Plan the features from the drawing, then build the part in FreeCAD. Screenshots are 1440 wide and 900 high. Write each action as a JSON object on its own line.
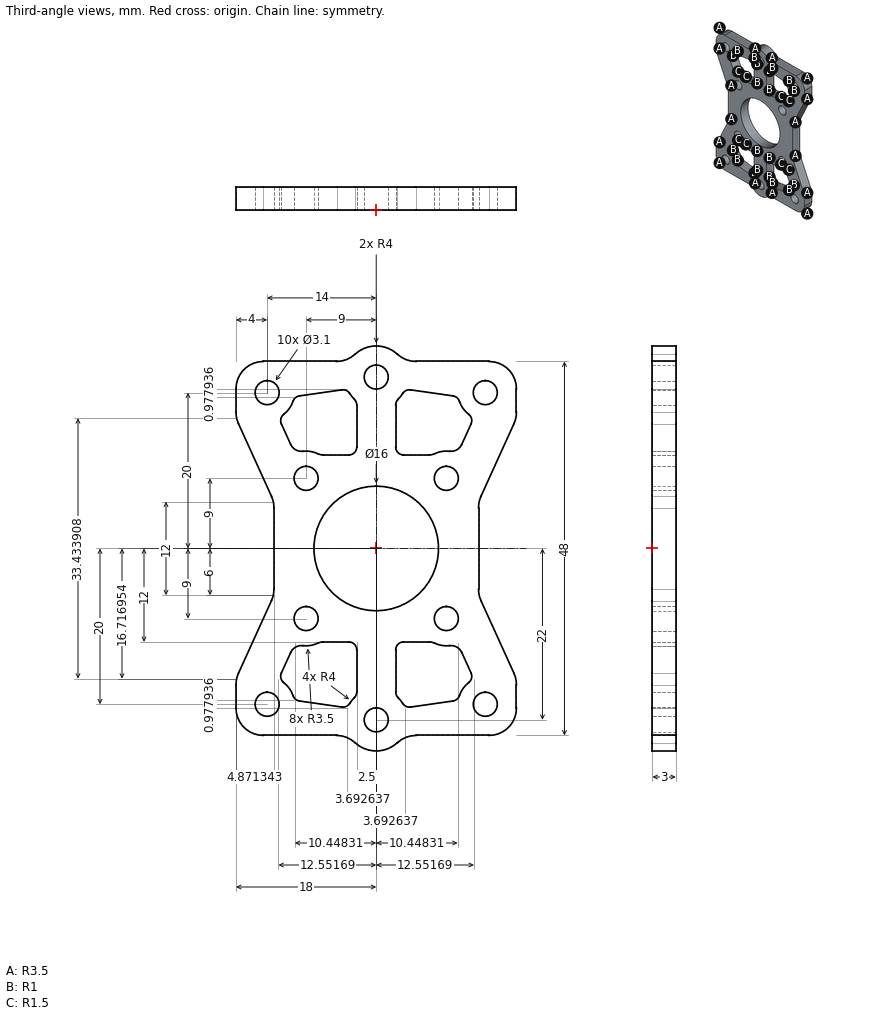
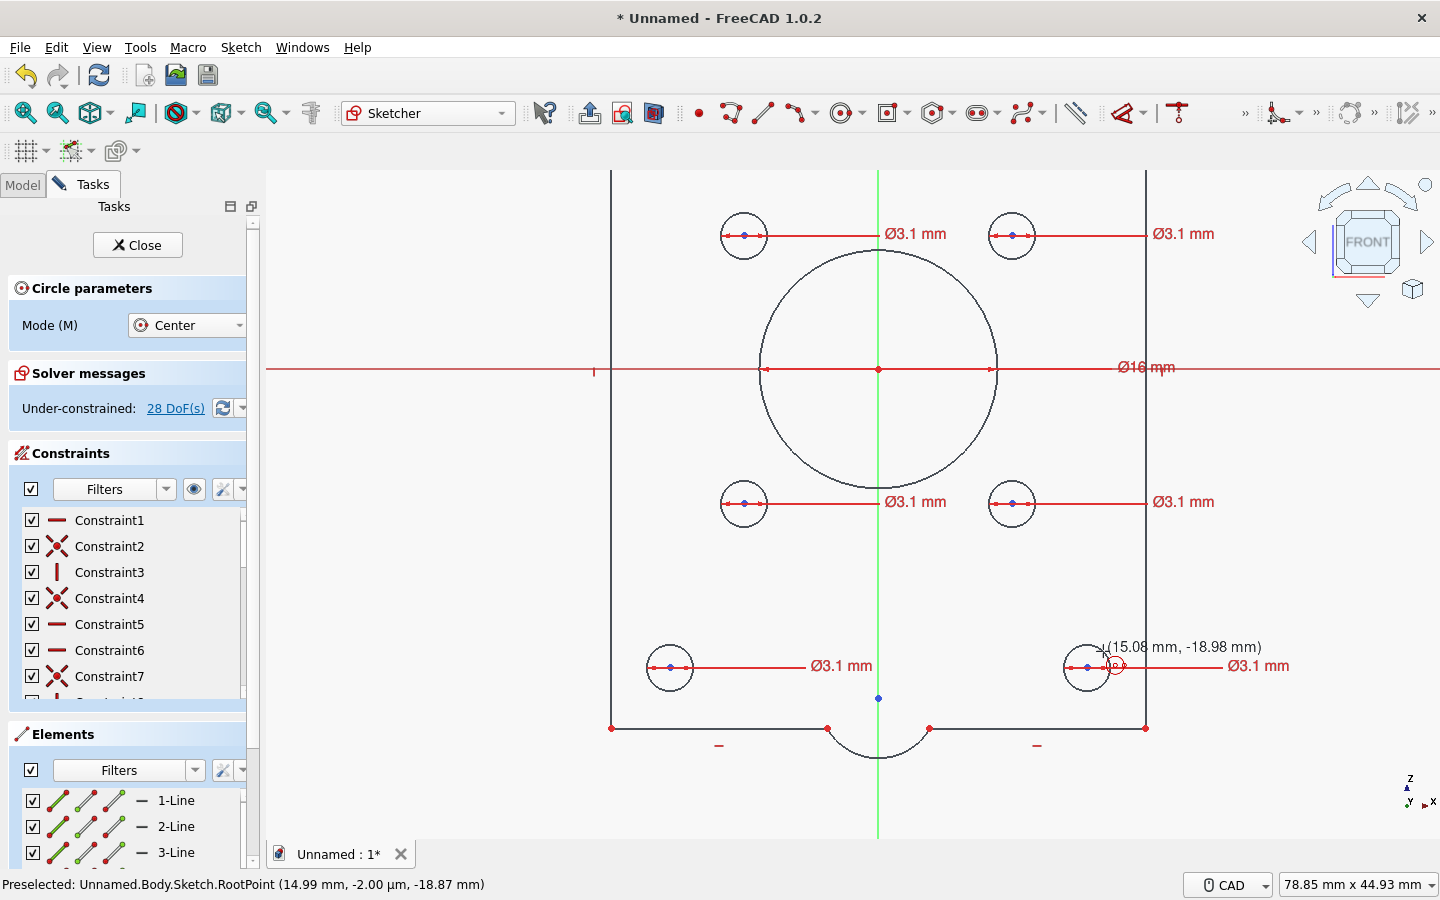
{"action": "left_click", "coordinate": [878, 697]}
{"action": "mouse_move", "coordinate": [895, 681]}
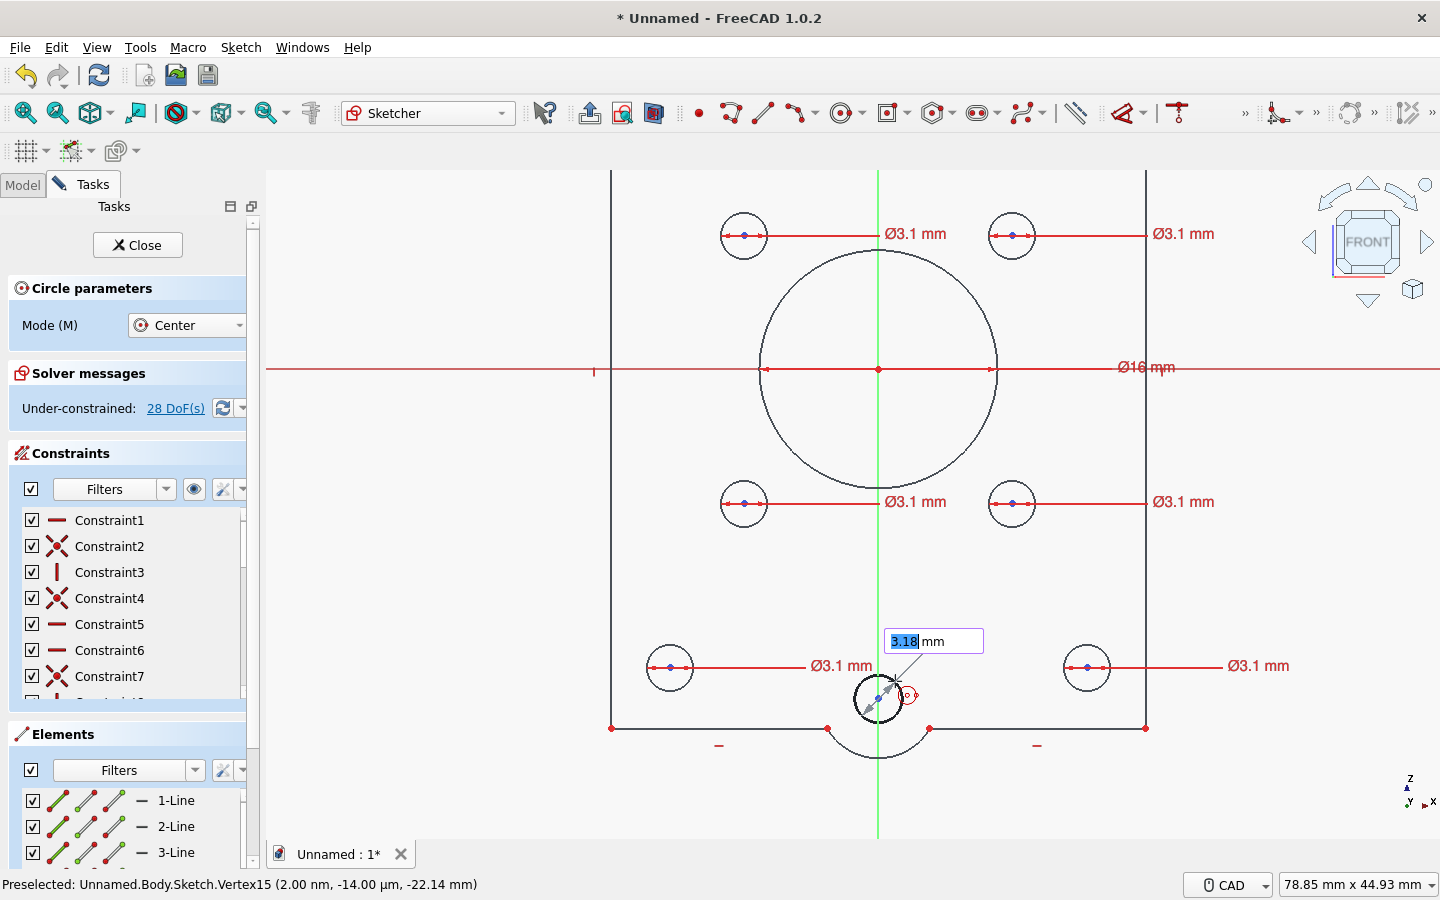
{"action": "type", "text": "3.1"}
{"action": "key", "text": "Return"}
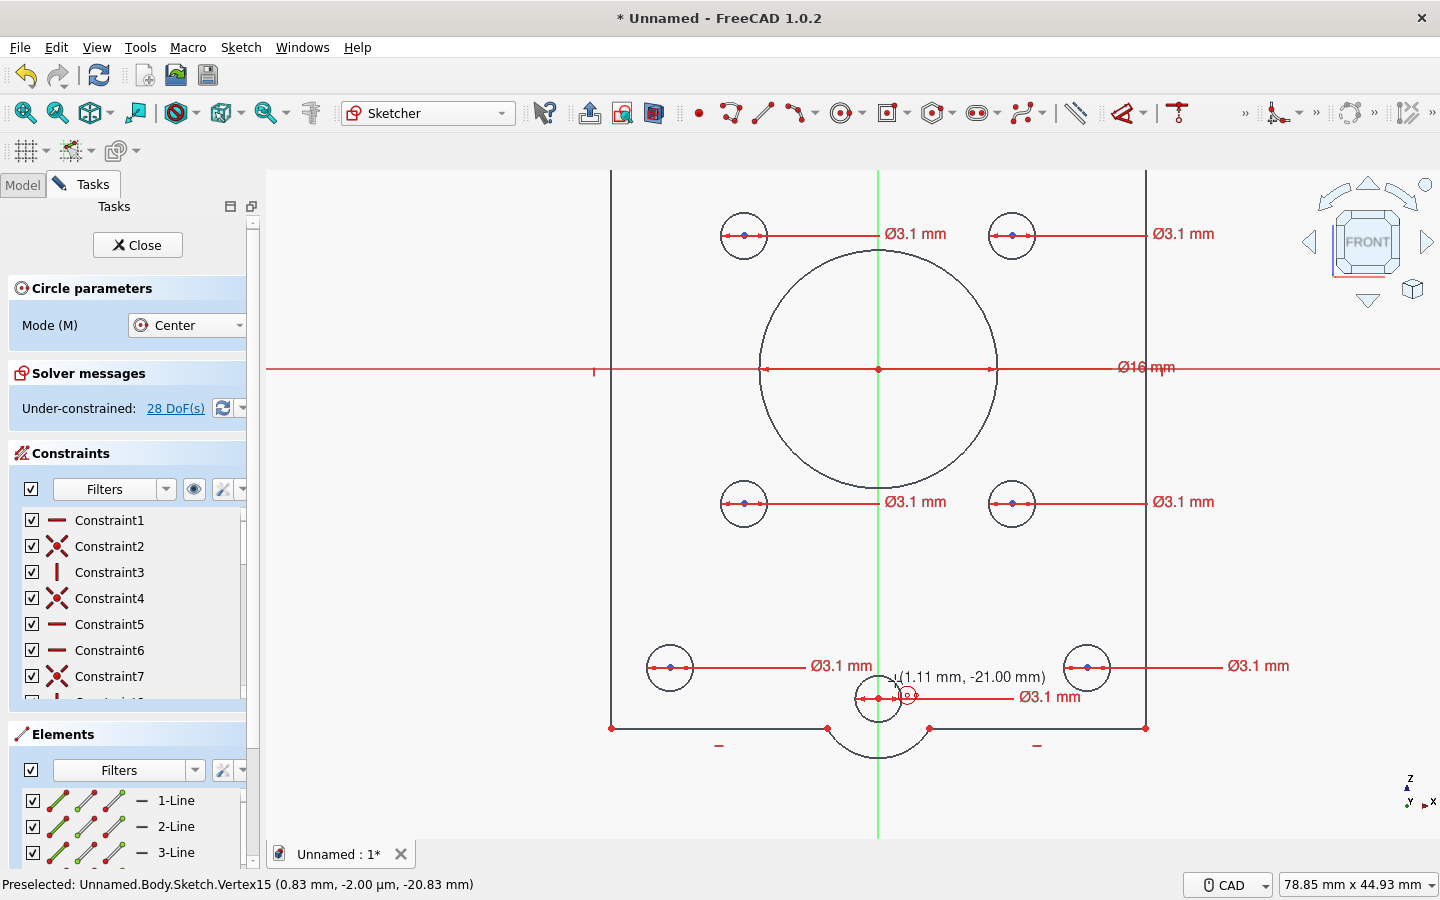
{"action": "scroll", "coordinate": [670, 669], "scroll_direction": "down", "scroll_amount": 3}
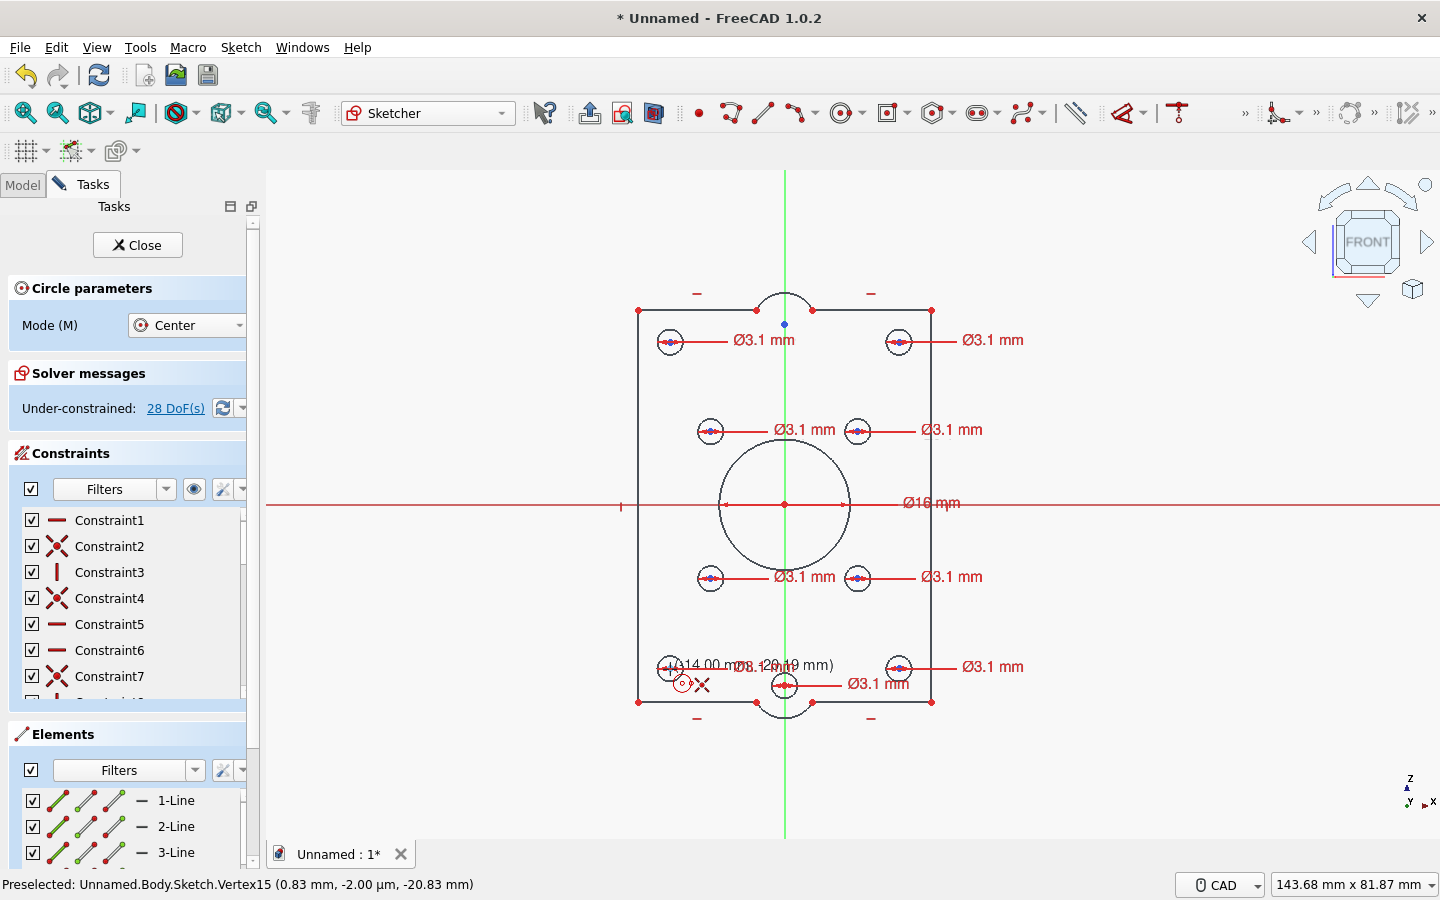
{"action": "scroll", "coordinate": [785, 325], "scroll_direction": "up", "scroll_amount": 3}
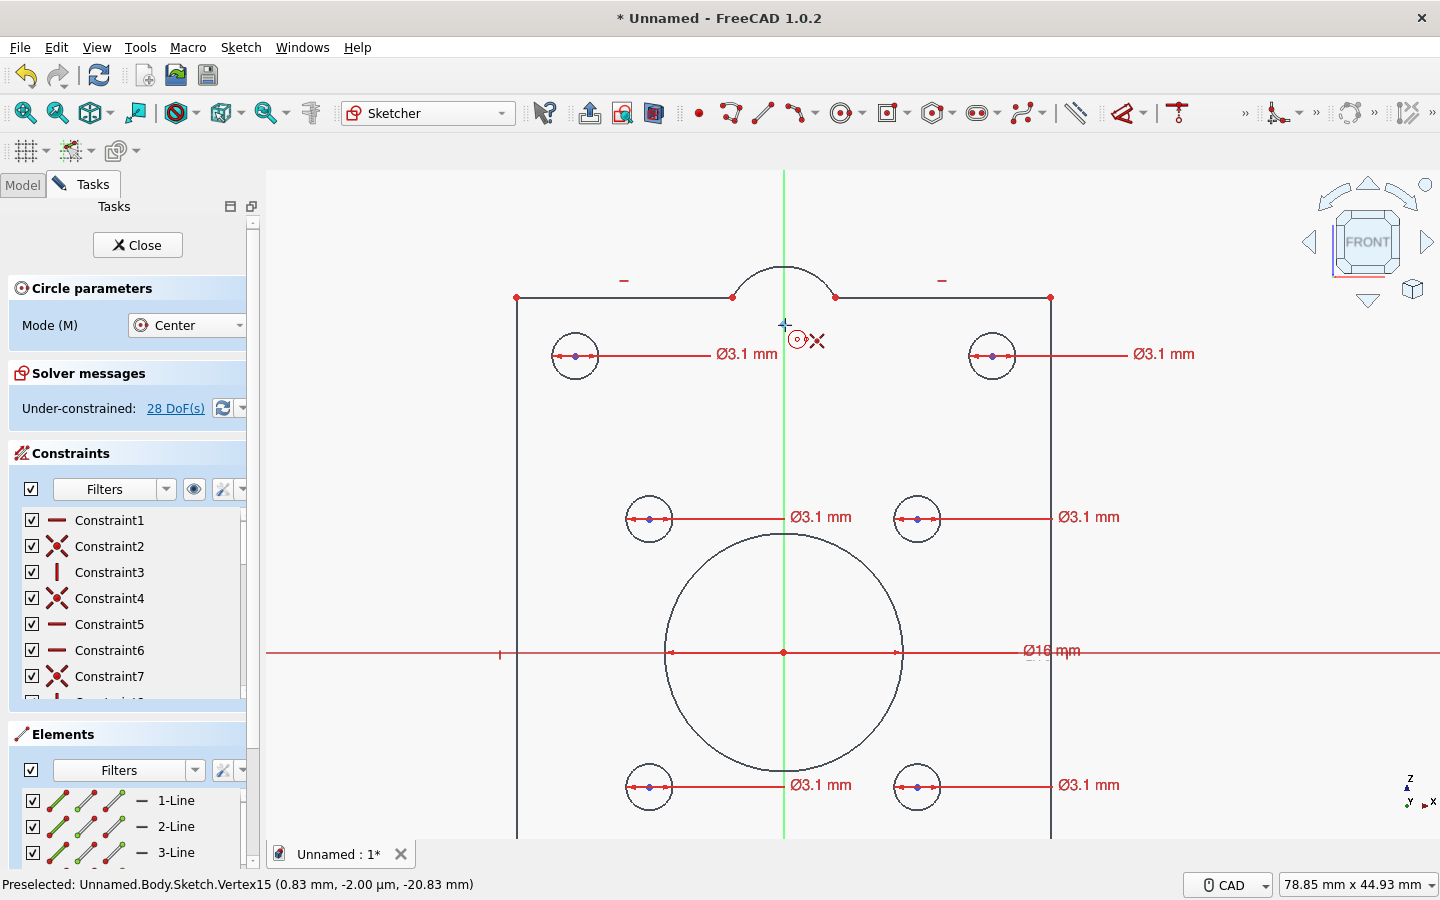
{"action": "left_click", "coordinate": [784, 325]}
{"action": "mouse_move", "coordinate": [800, 309]}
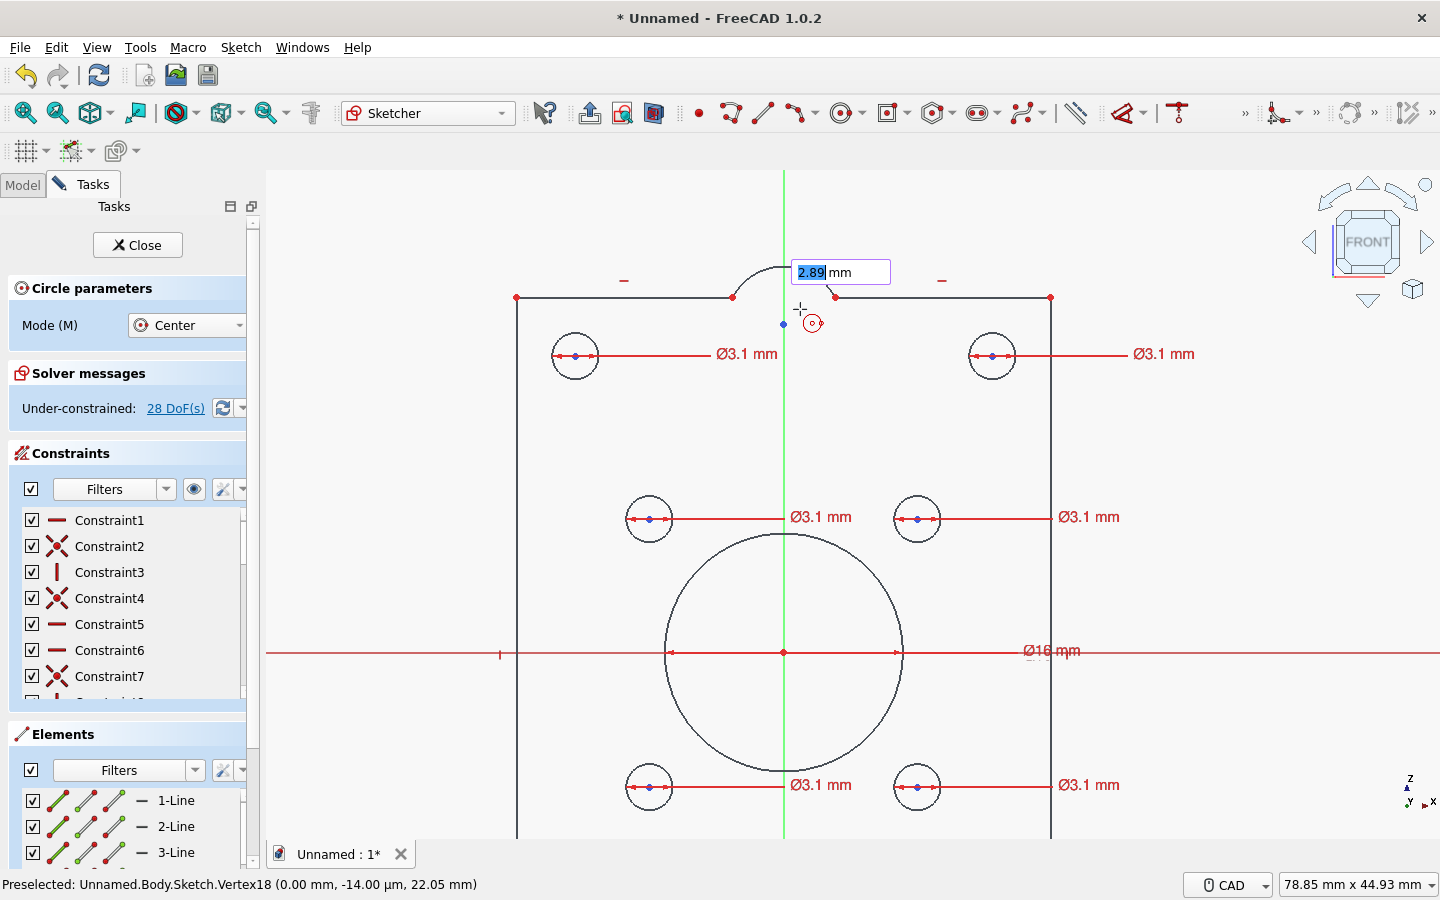
{"action": "type", "text": "3.1"}
{"action": "key", "text": "Return"}
{"action": "key", "text": "Escape"}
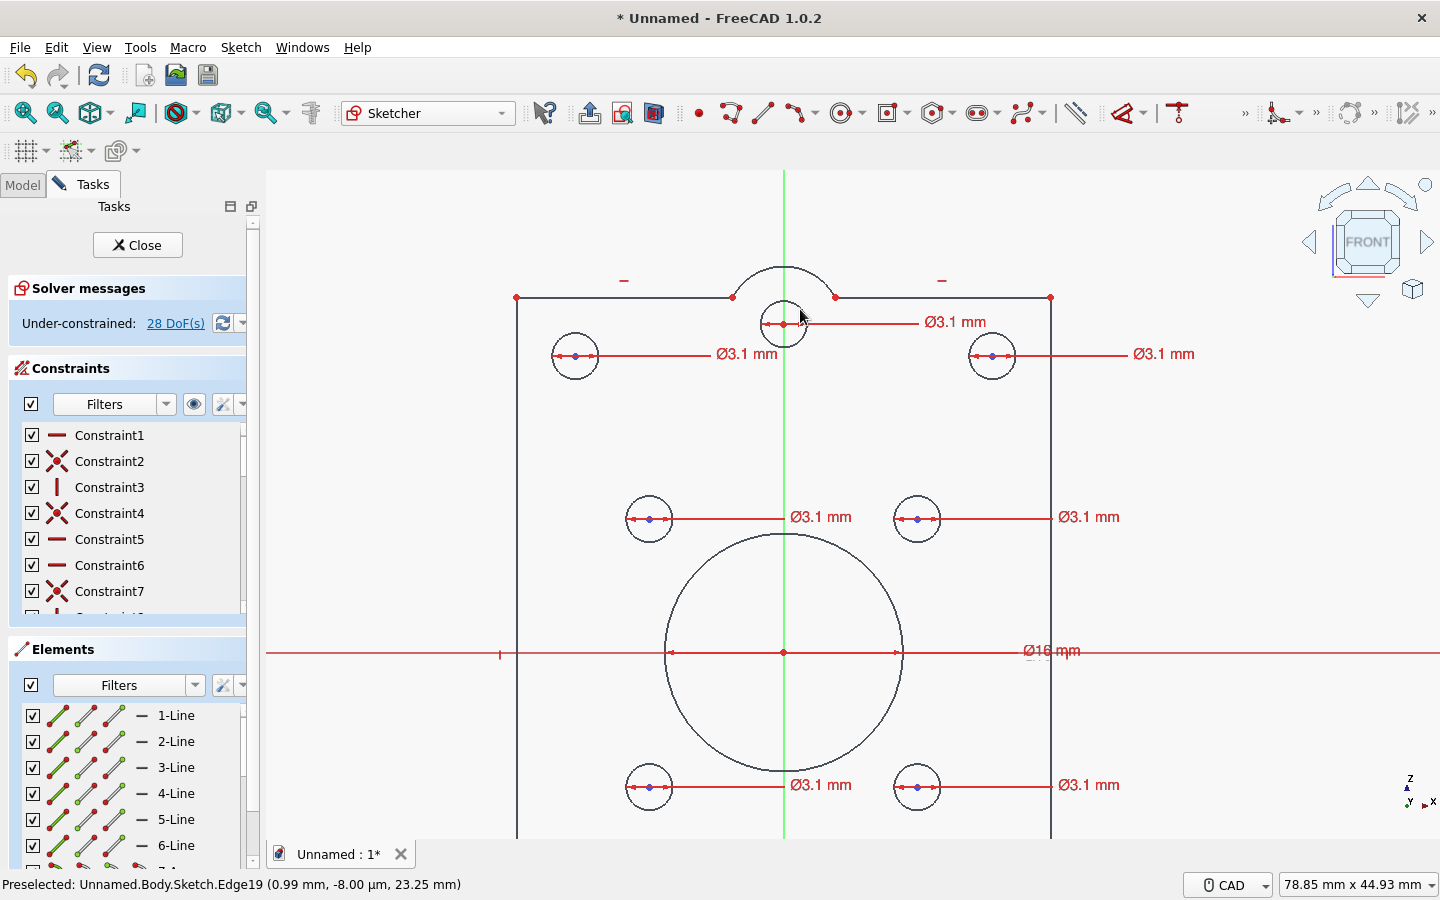
{"action": "scroll", "coordinate": [785, 324], "scroll_direction": "down", "scroll_amount": 3}